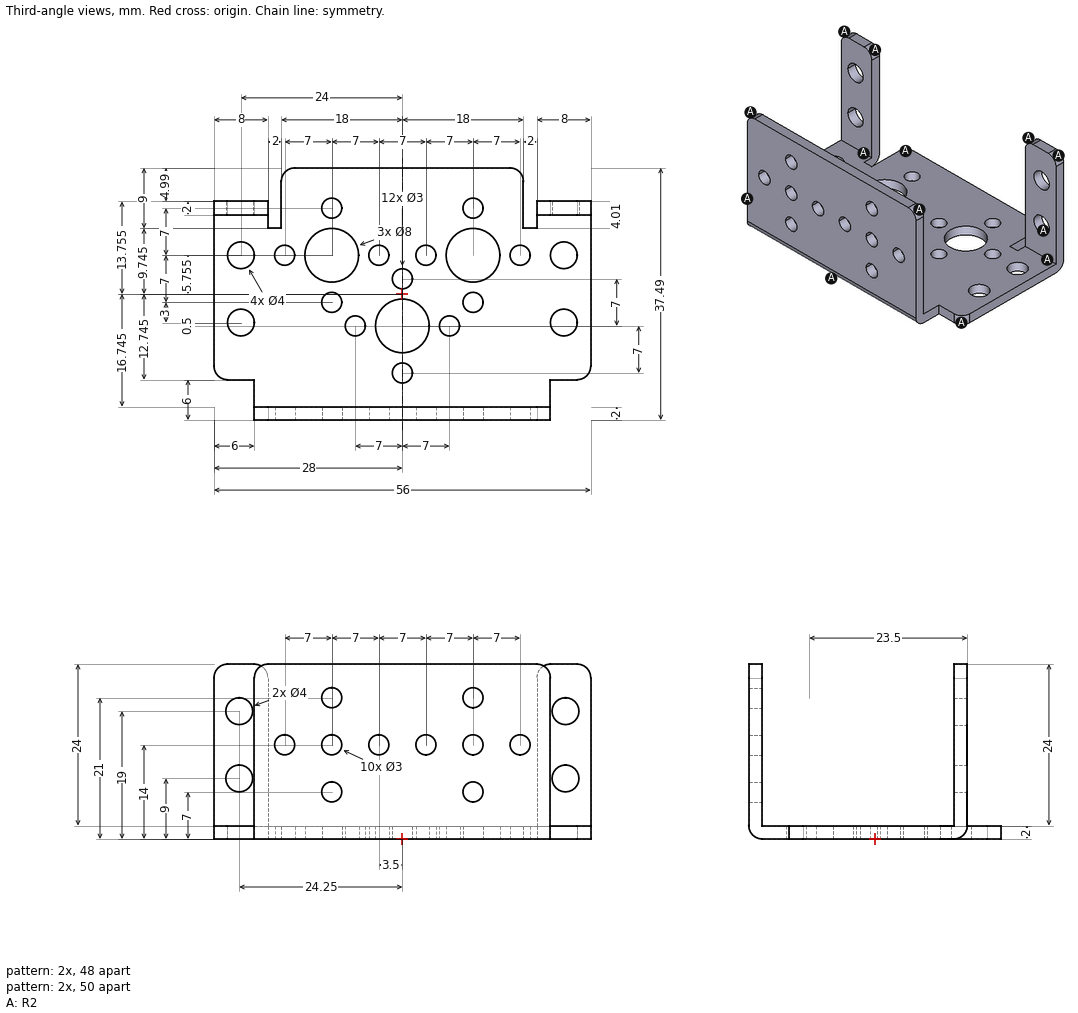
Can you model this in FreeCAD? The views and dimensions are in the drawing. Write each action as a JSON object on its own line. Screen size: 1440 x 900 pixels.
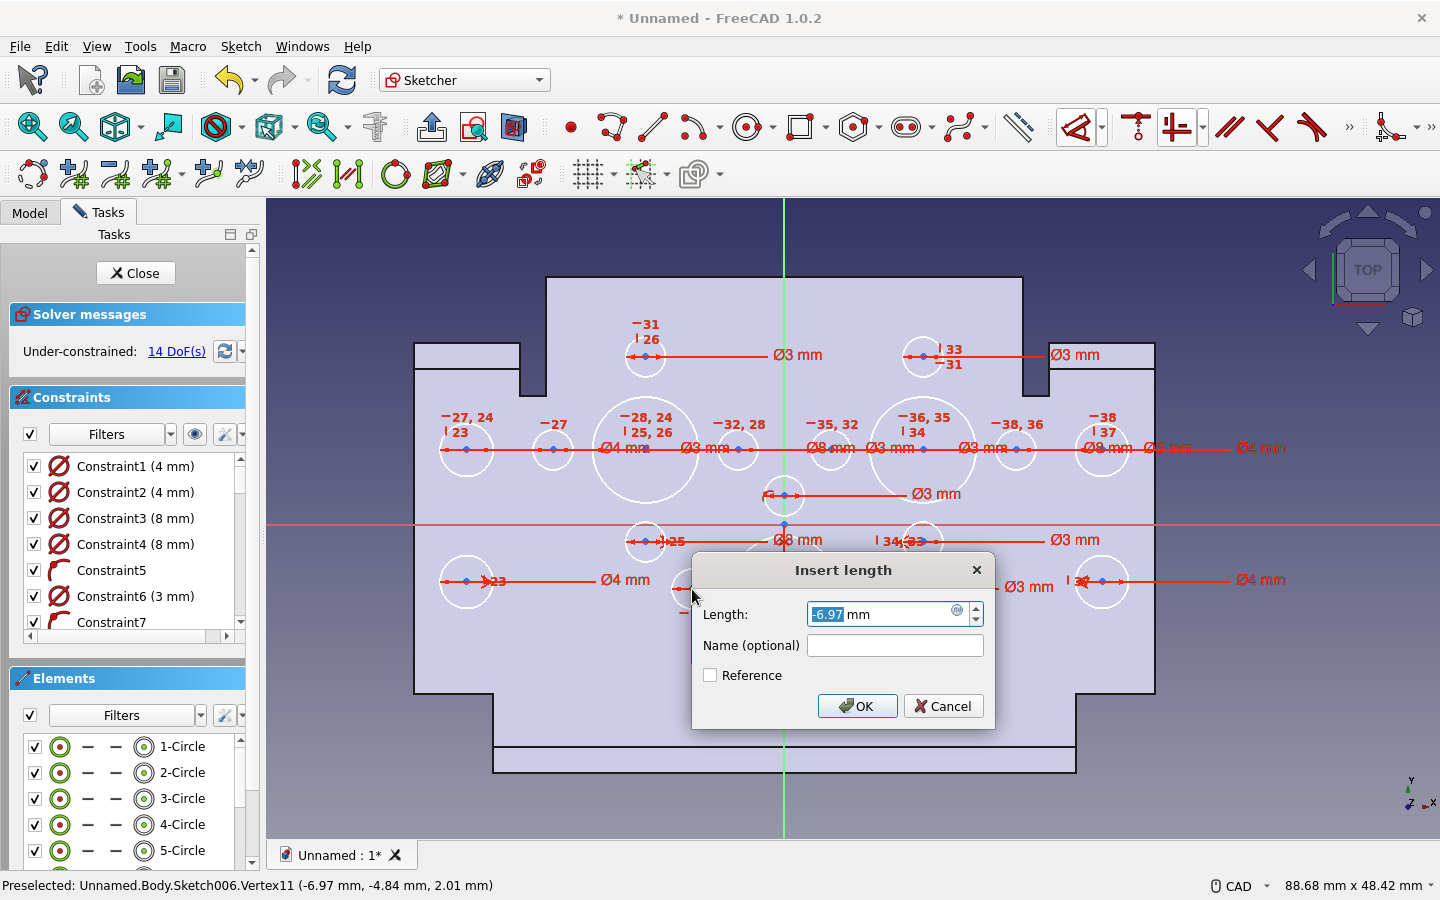
{"action": "type", "text": "-7"}
{"action": "key", "text": "Return"}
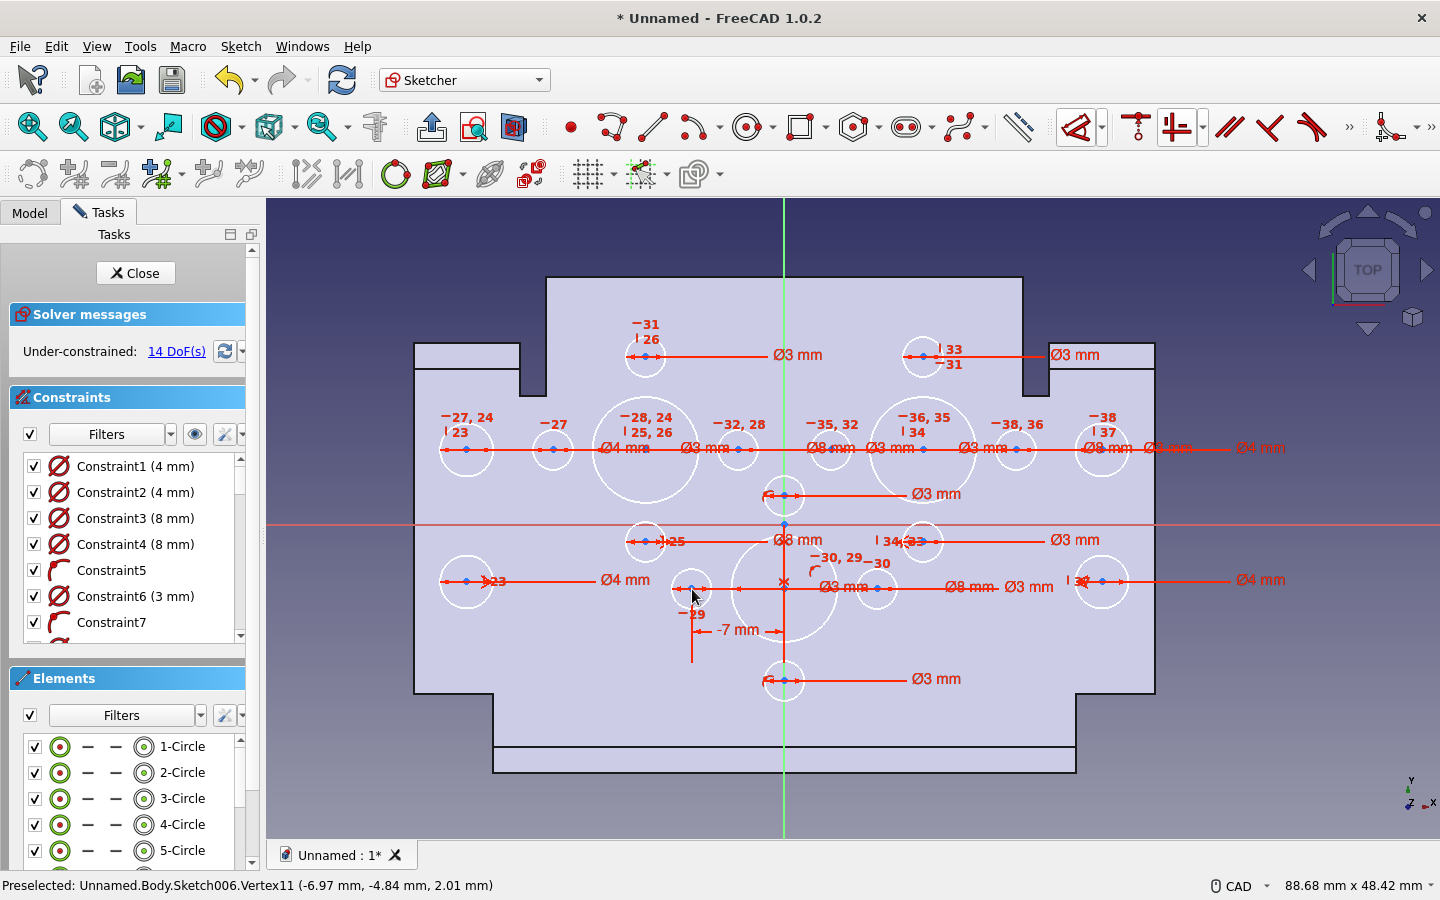
{"action": "left_click", "coordinate": [877, 589]}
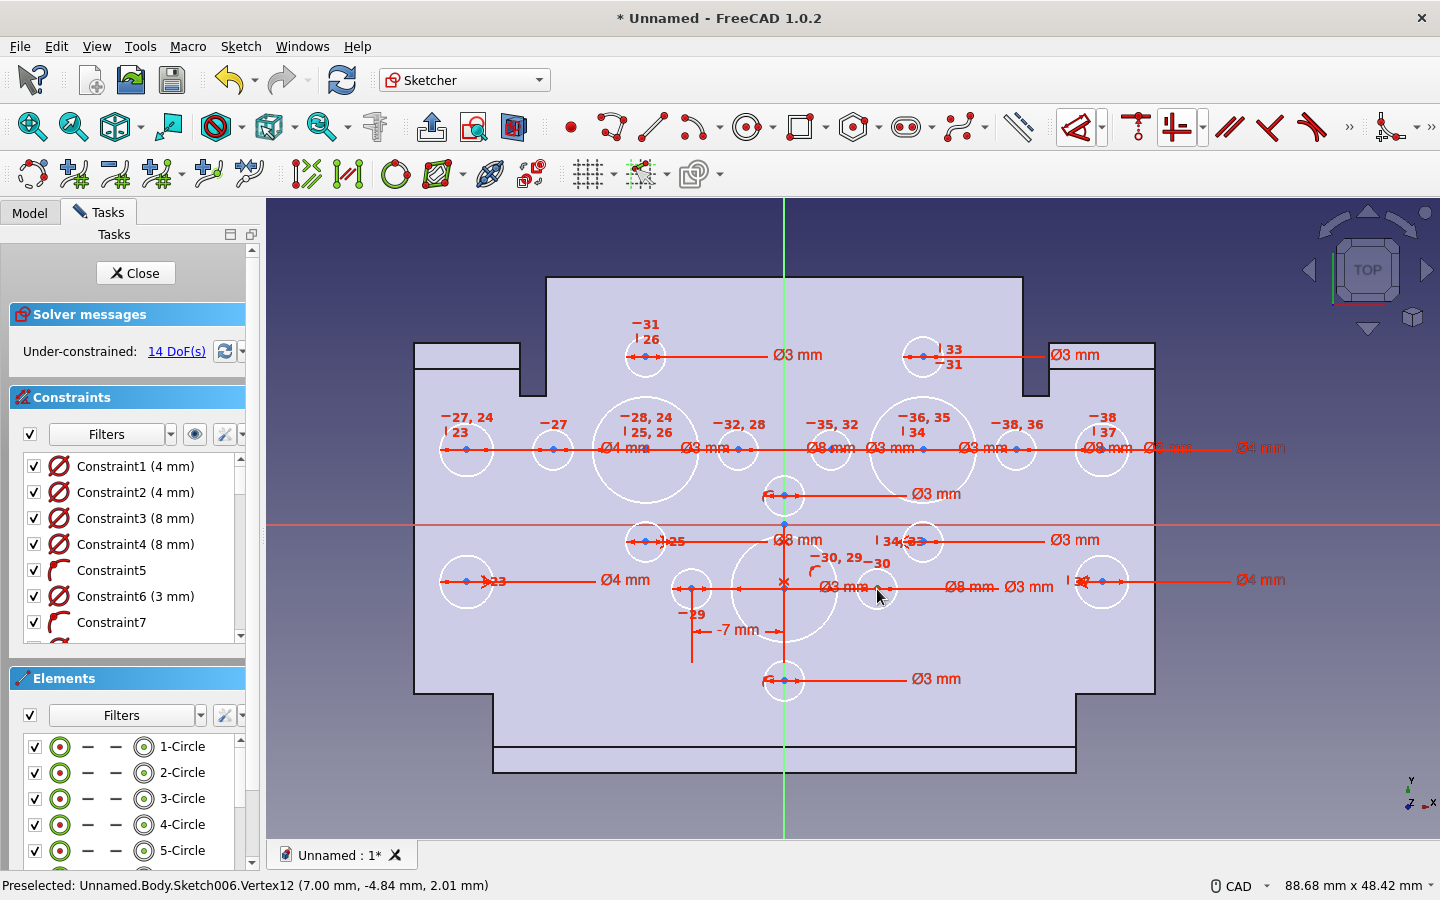
{"action": "left_click", "coordinate": [1102, 128]}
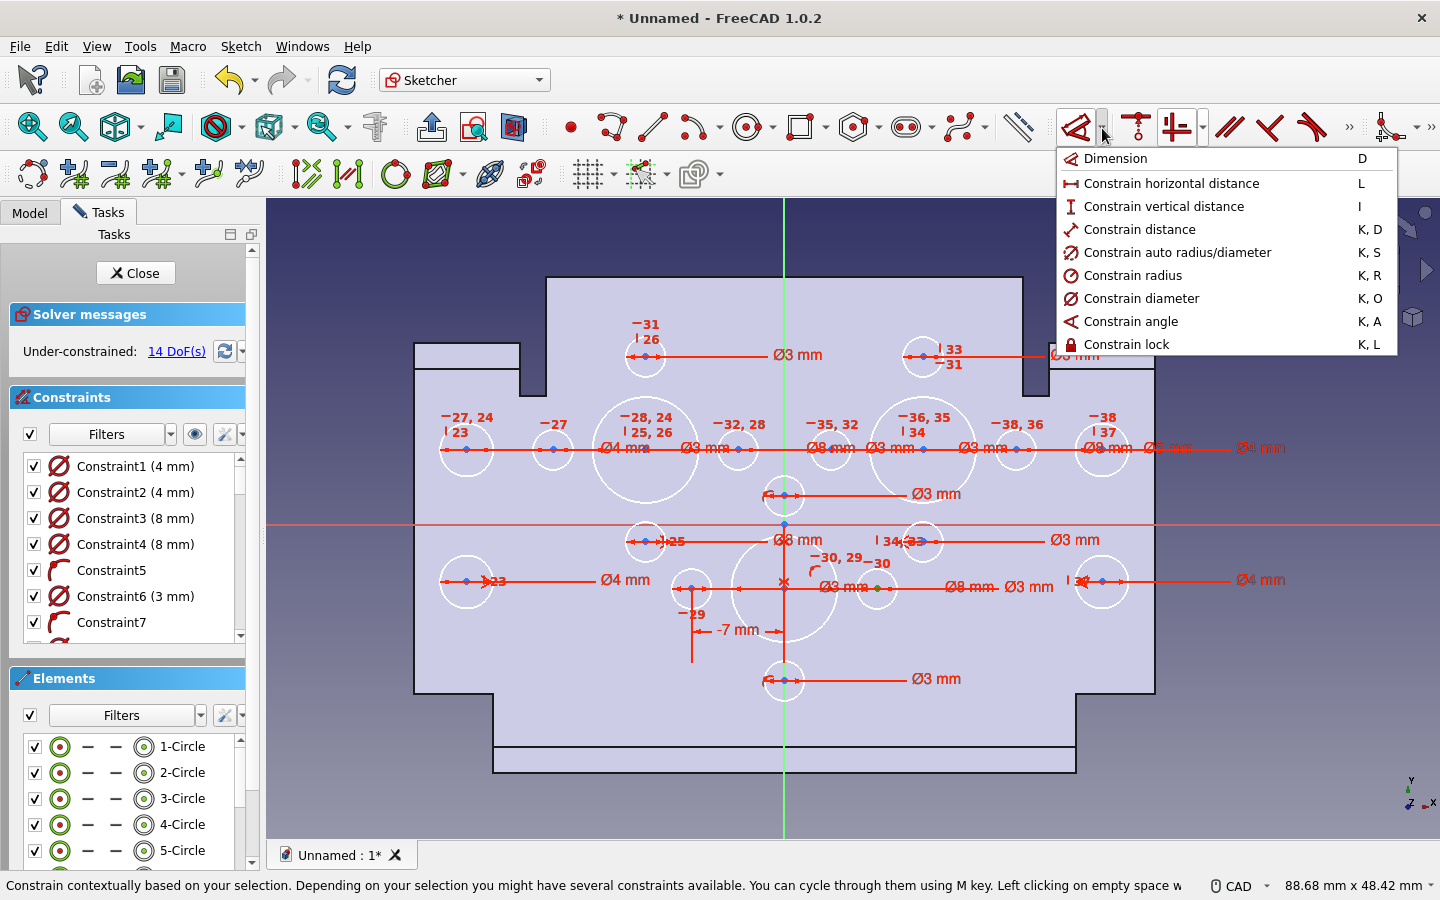
{"action": "left_click", "coordinate": [1227, 184]}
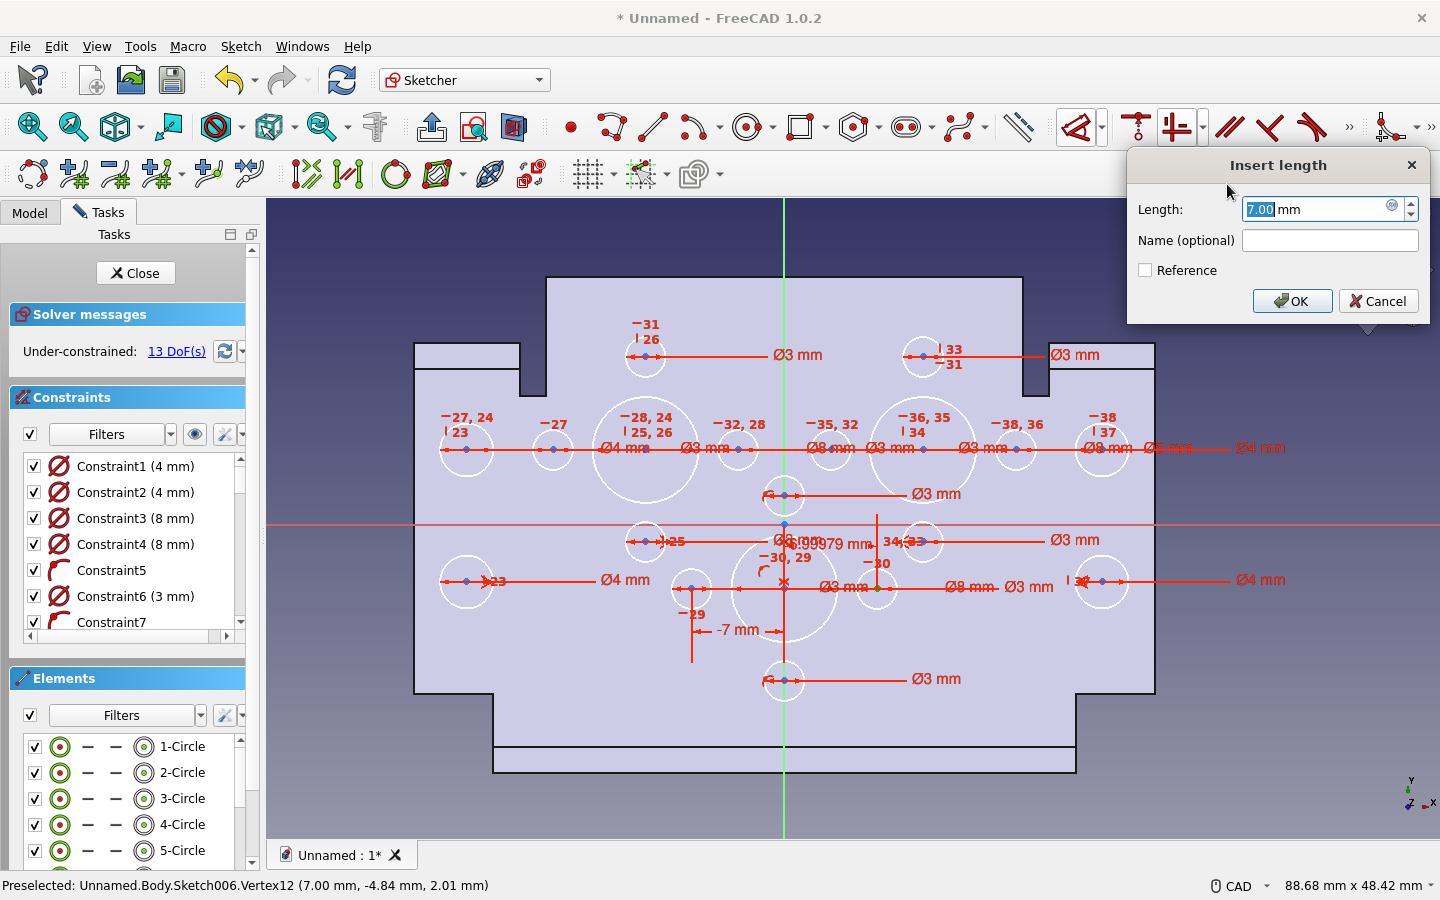
{"action": "type", "text": "7"}
{"action": "key", "text": "Return"}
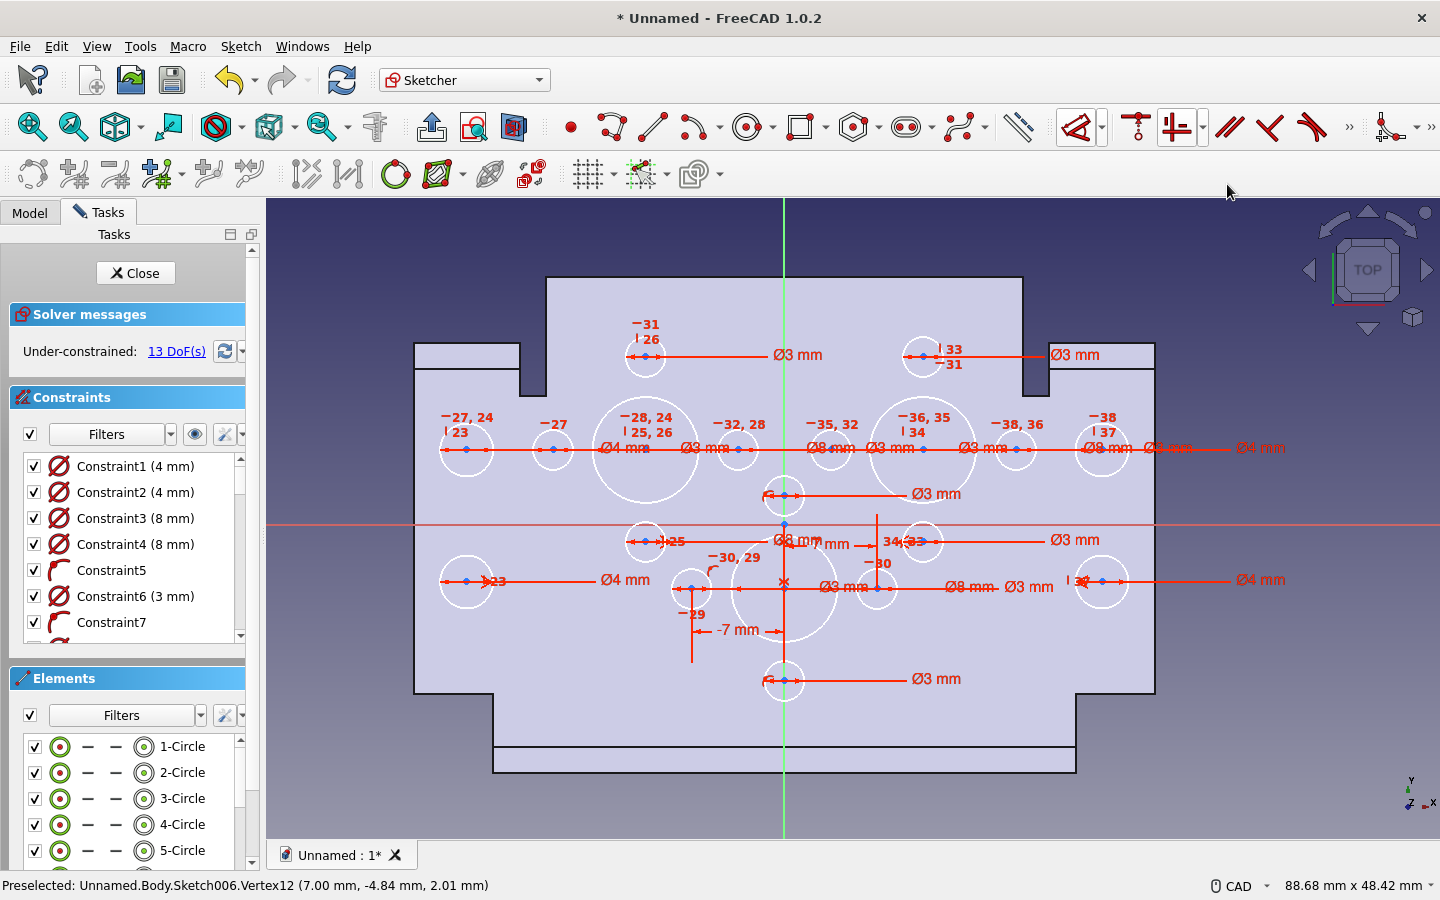
{"action": "left_click", "coordinate": [467, 450]}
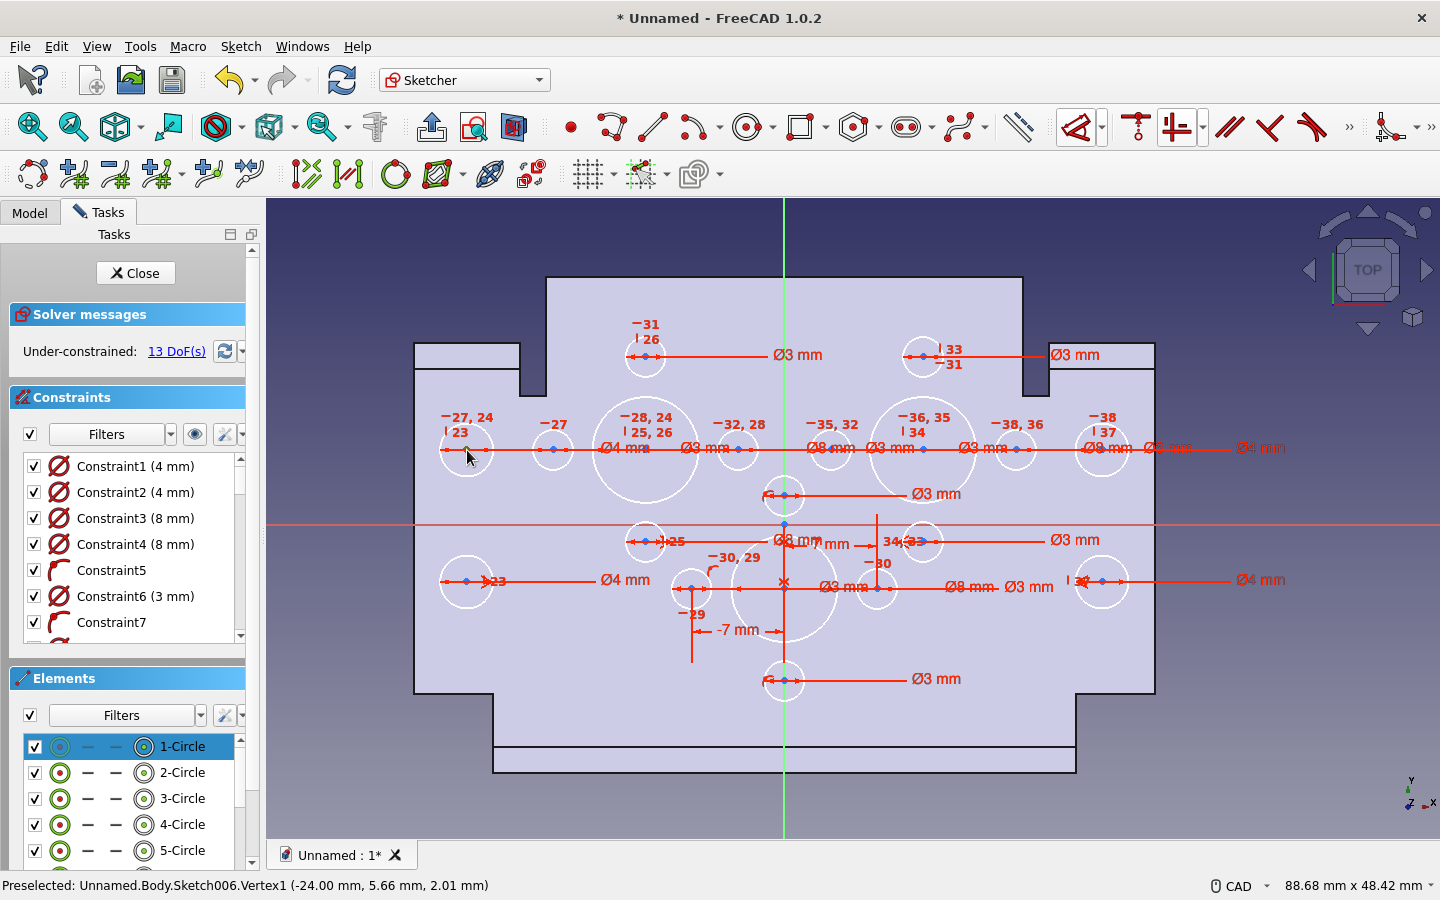
{"action": "key", "text": "l"}